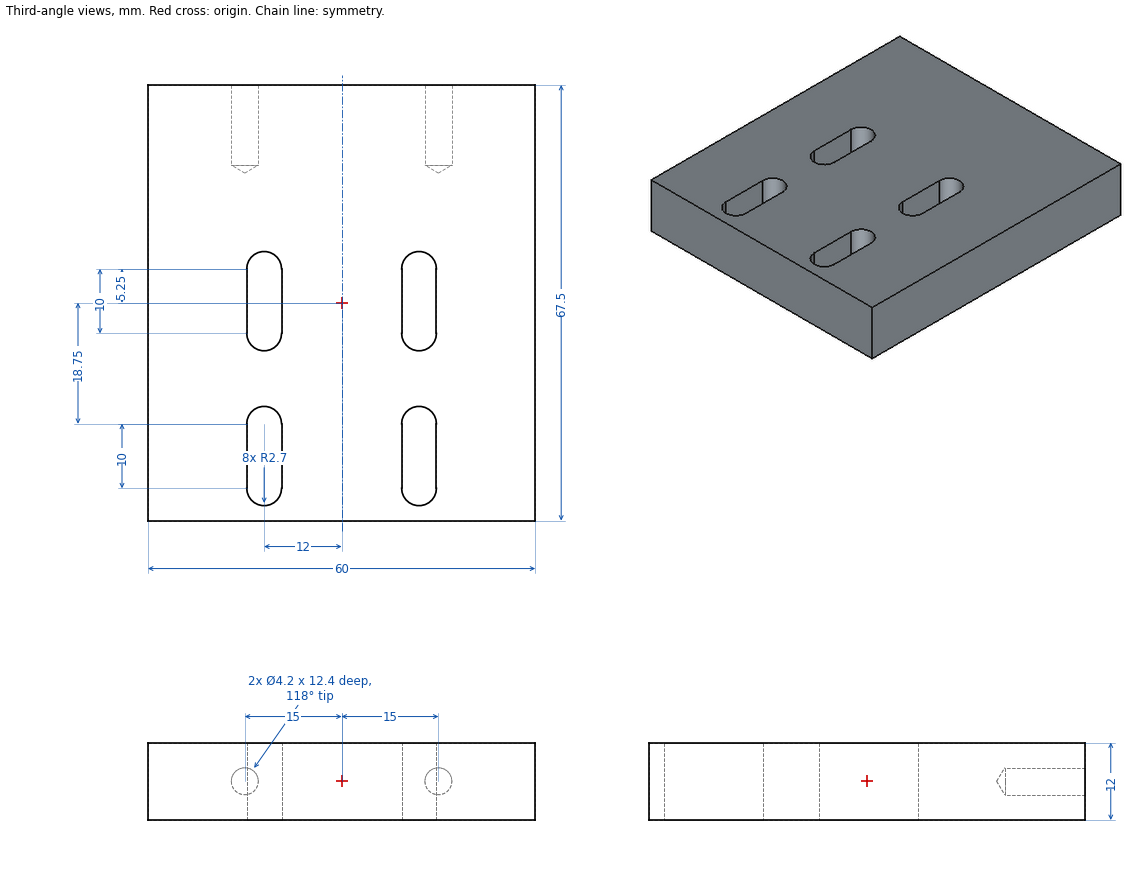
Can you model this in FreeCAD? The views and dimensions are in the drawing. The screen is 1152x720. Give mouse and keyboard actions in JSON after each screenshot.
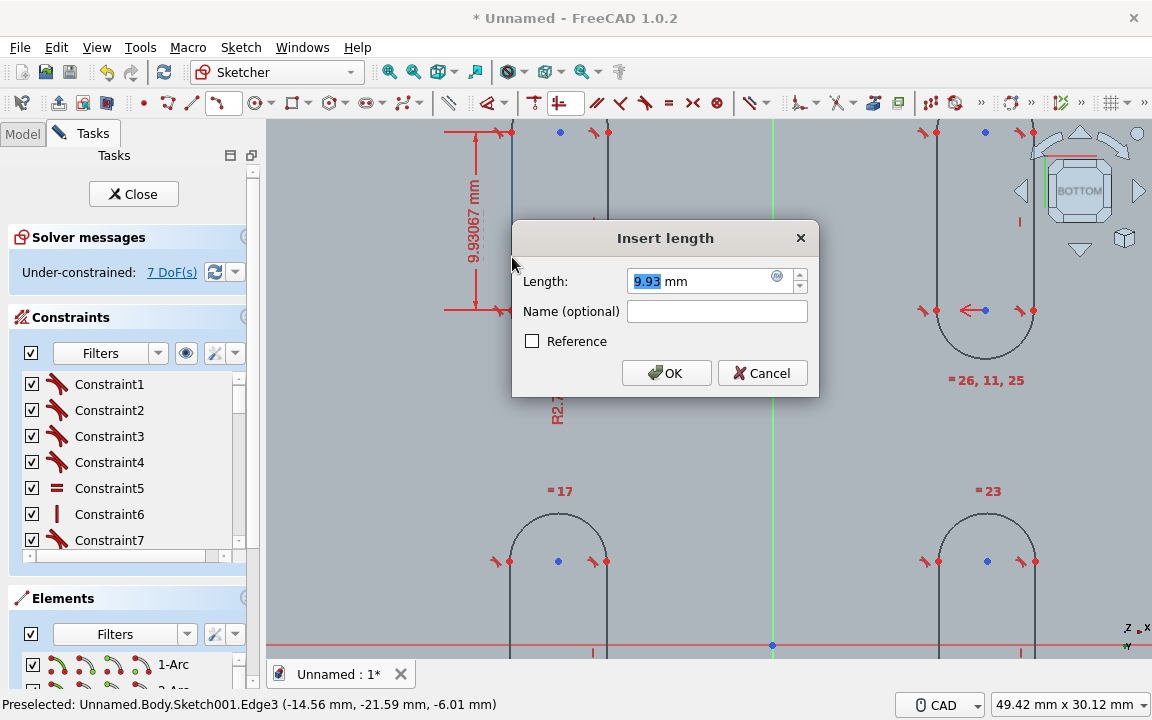
{"action": "type", "text": "10"}
{"action": "key", "text": "Return"}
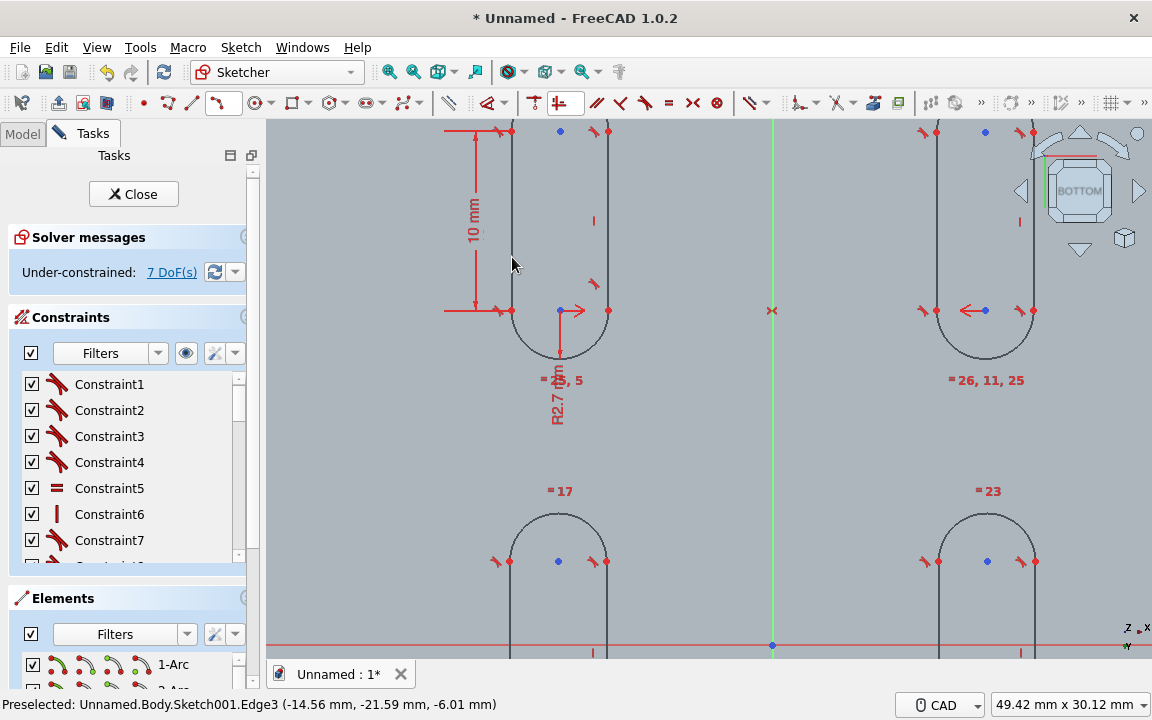
{"action": "left_click", "coordinate": [937, 257]}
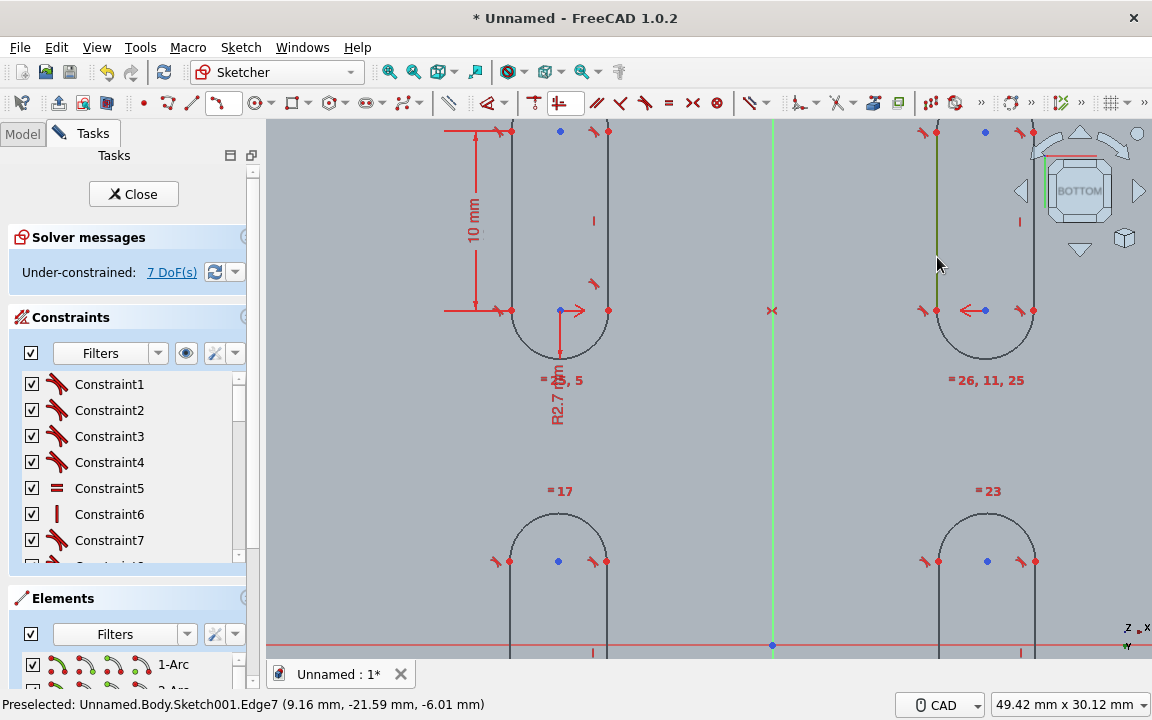
{"action": "key", "text": "i"}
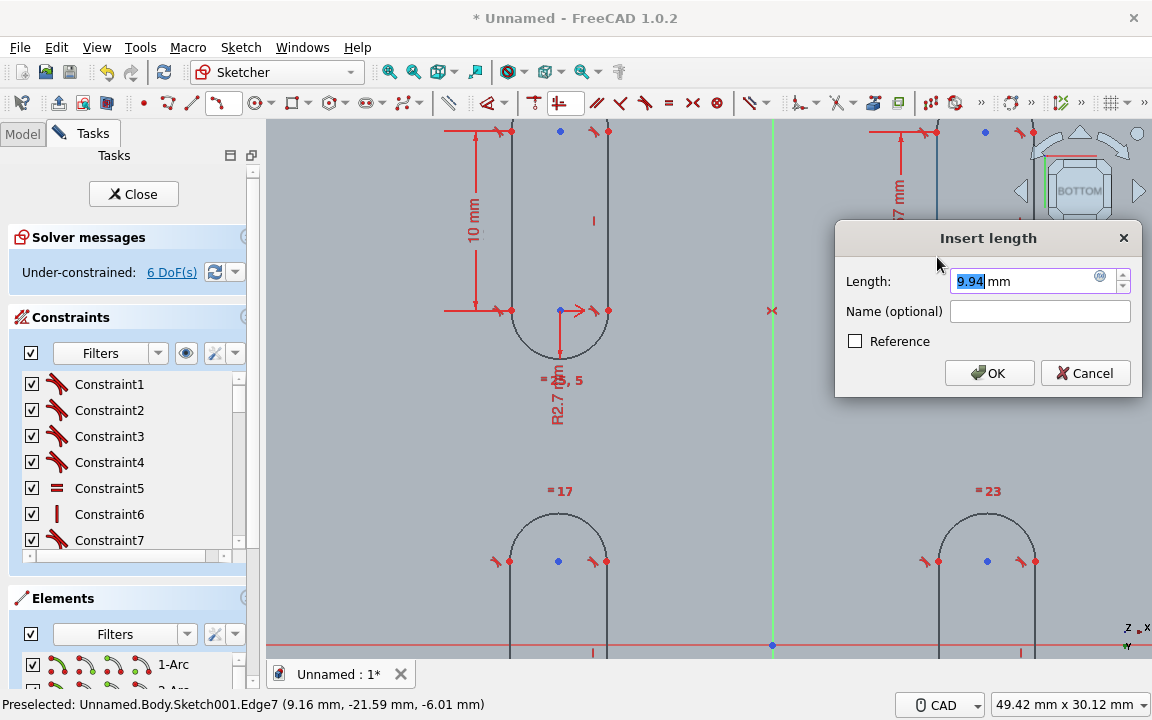
{"action": "type", "text": "10"}
{"action": "key", "text": "Return"}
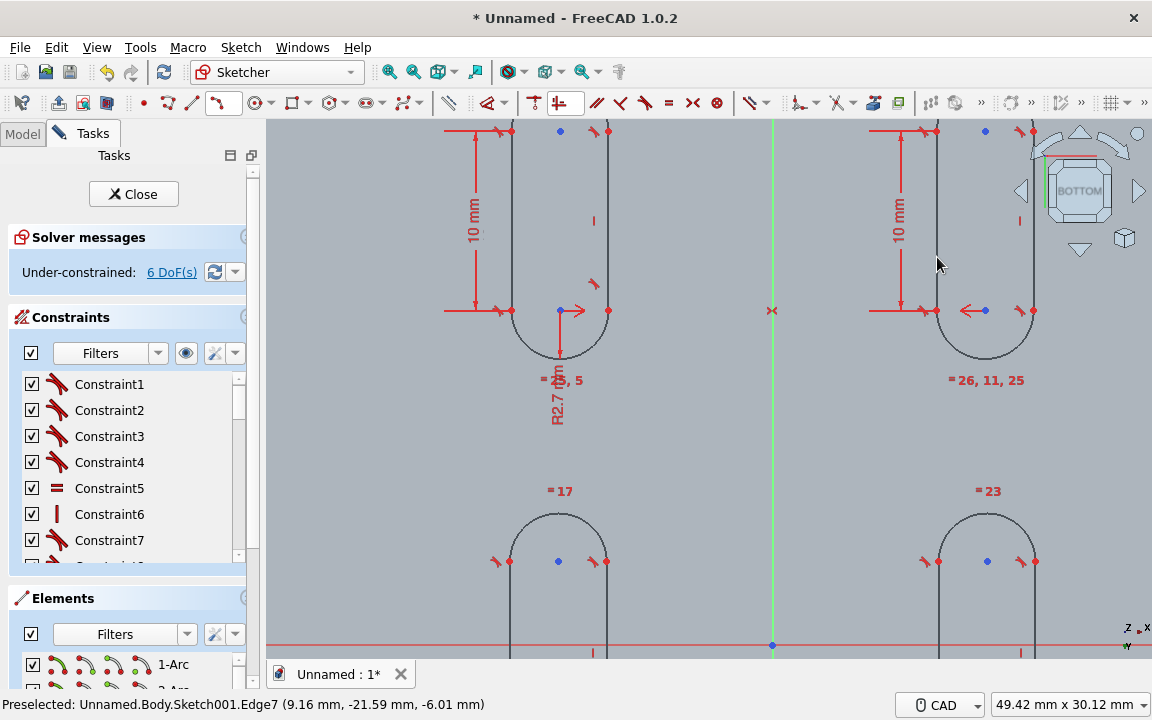
{"action": "left_click", "coordinate": [510, 616]}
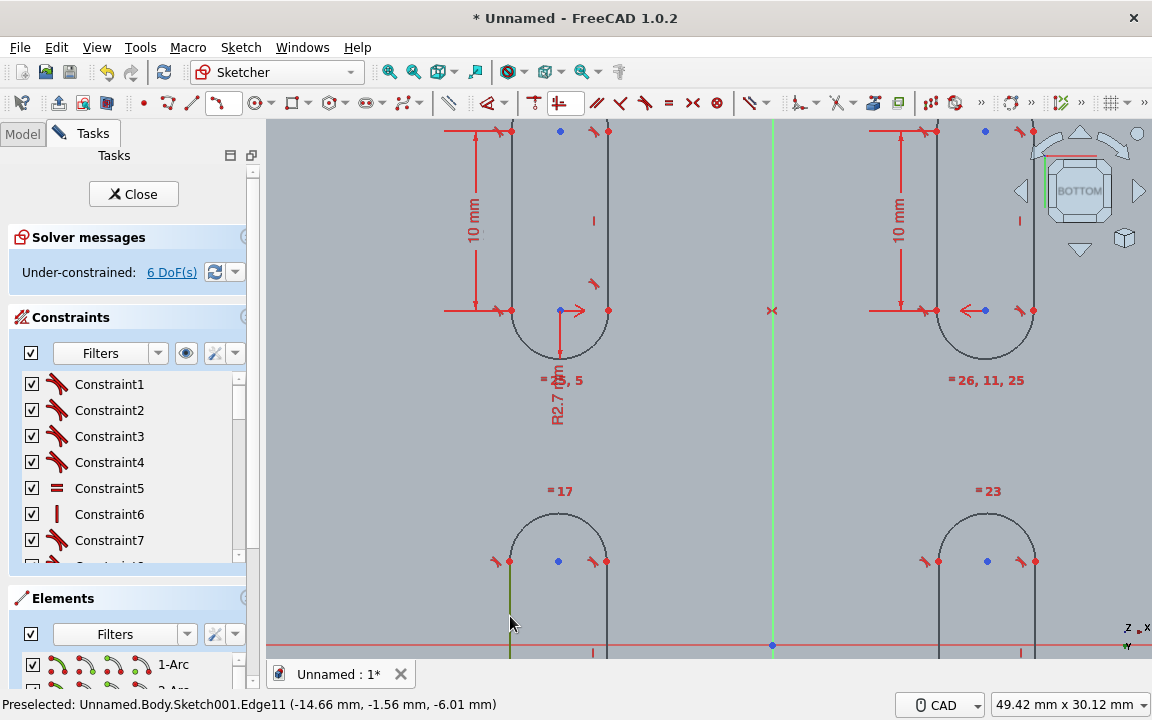
{"action": "left_click", "coordinate": [506, 104]}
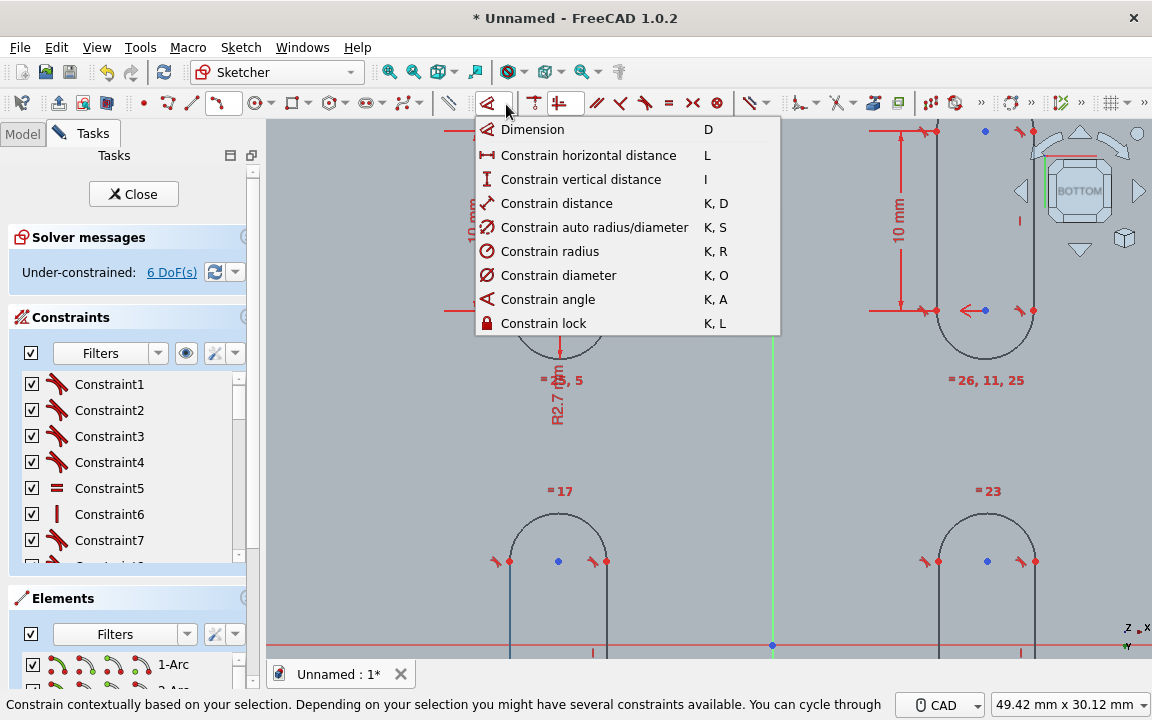
{"action": "left_click", "coordinate": [628, 179]}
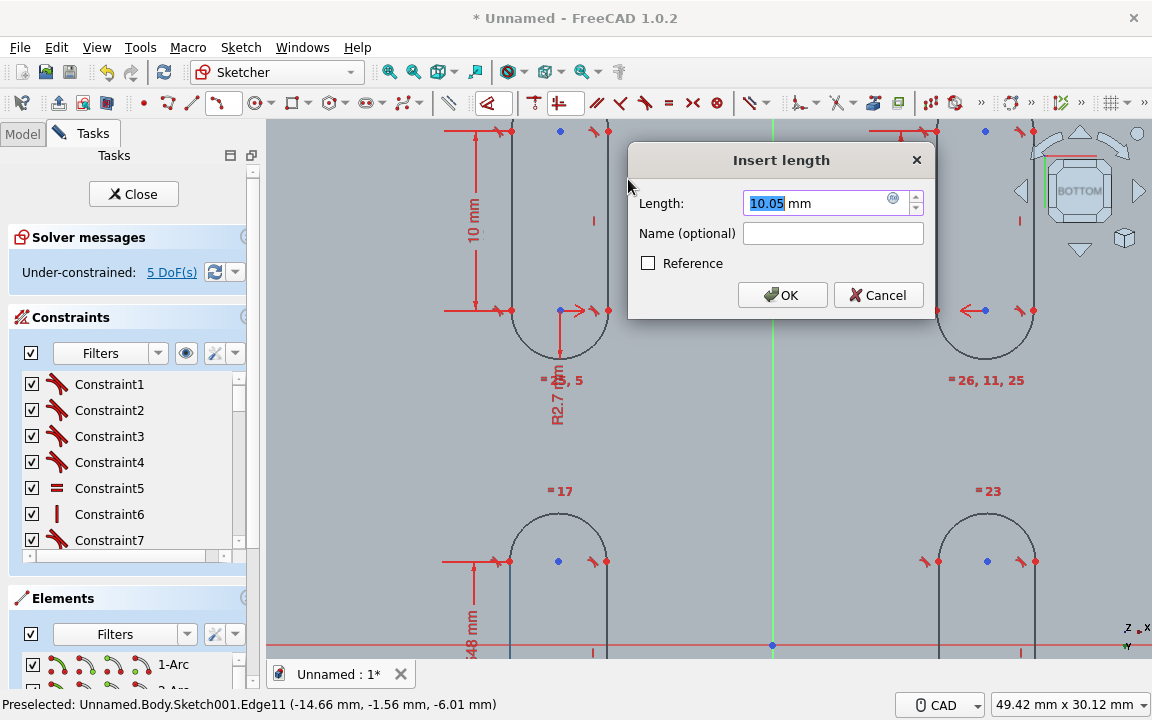
{"action": "type", "text": "10"}
{"action": "key", "text": "Return"}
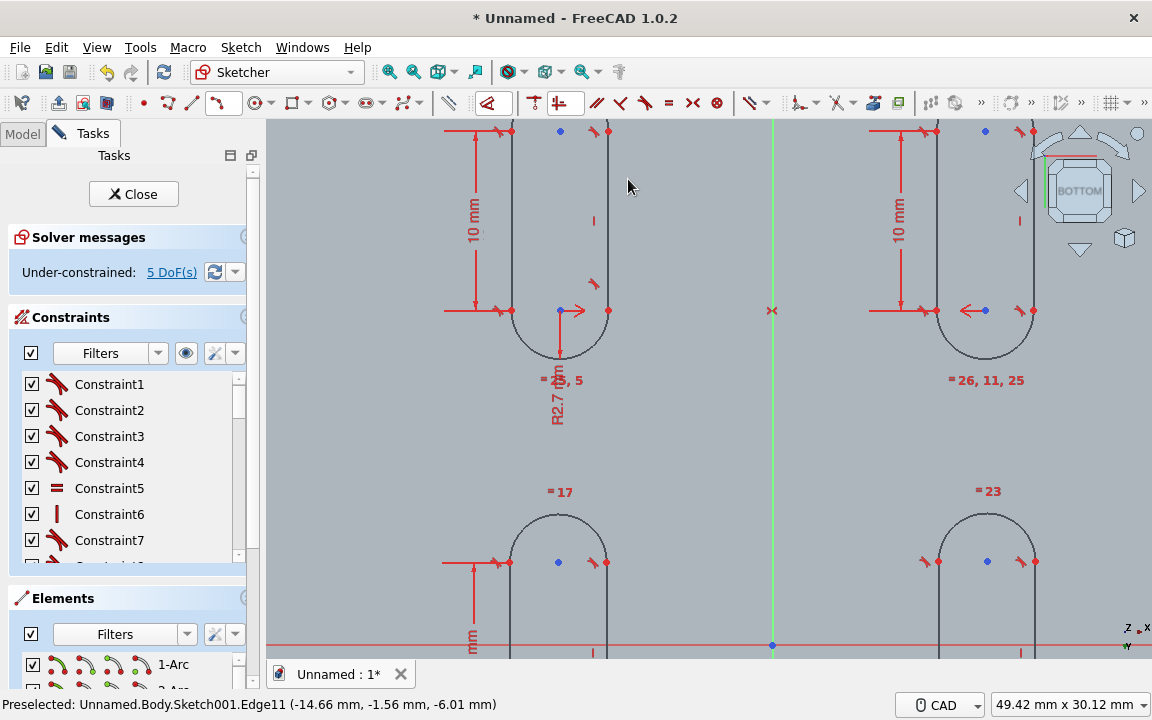
{"action": "left_click", "coordinate": [939, 616]}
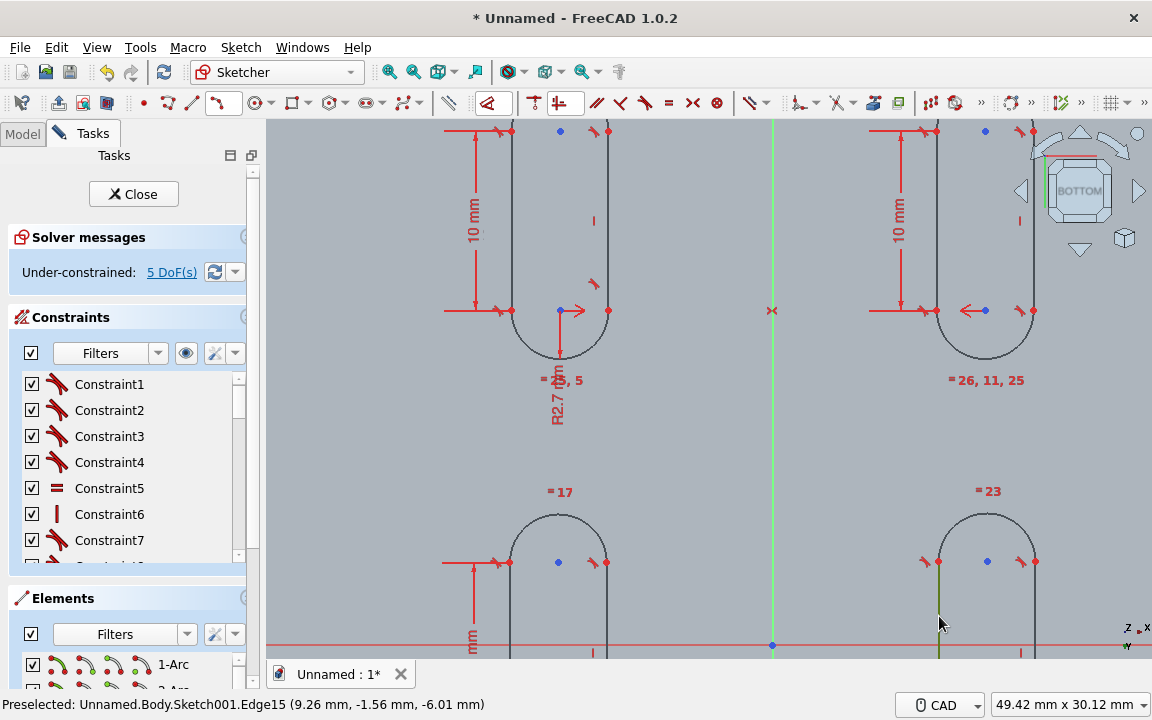
{"action": "key", "text": "i"}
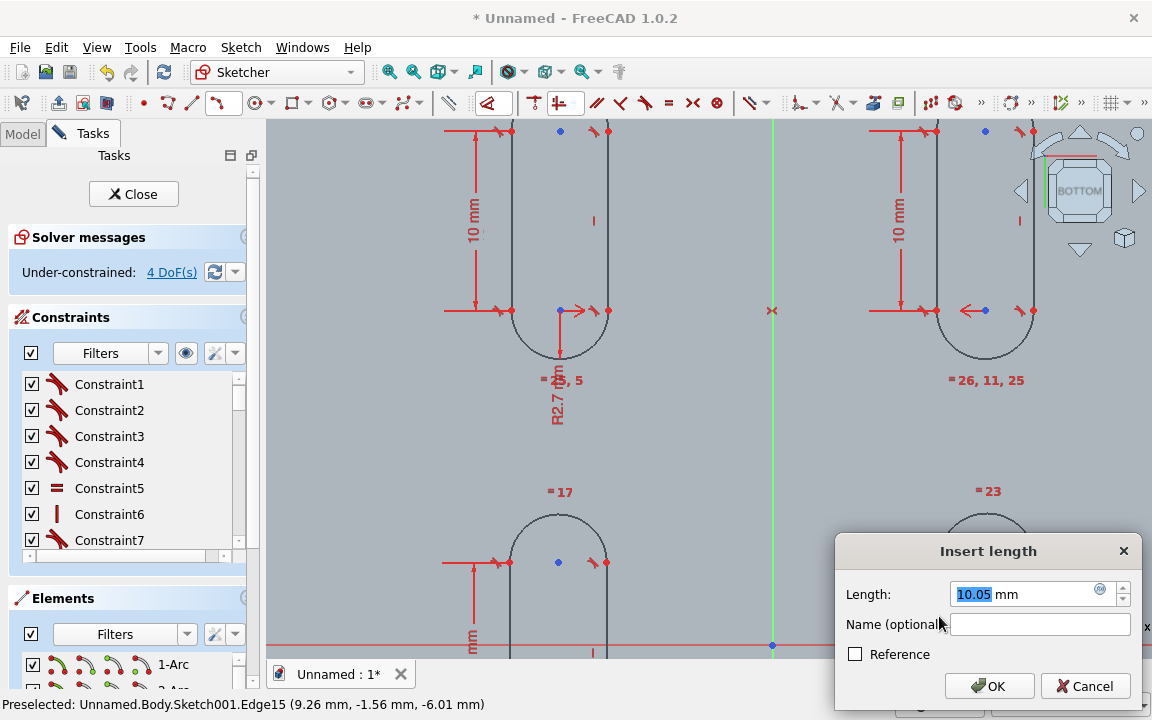
{"action": "type", "text": "10"}
{"action": "key", "text": "Return"}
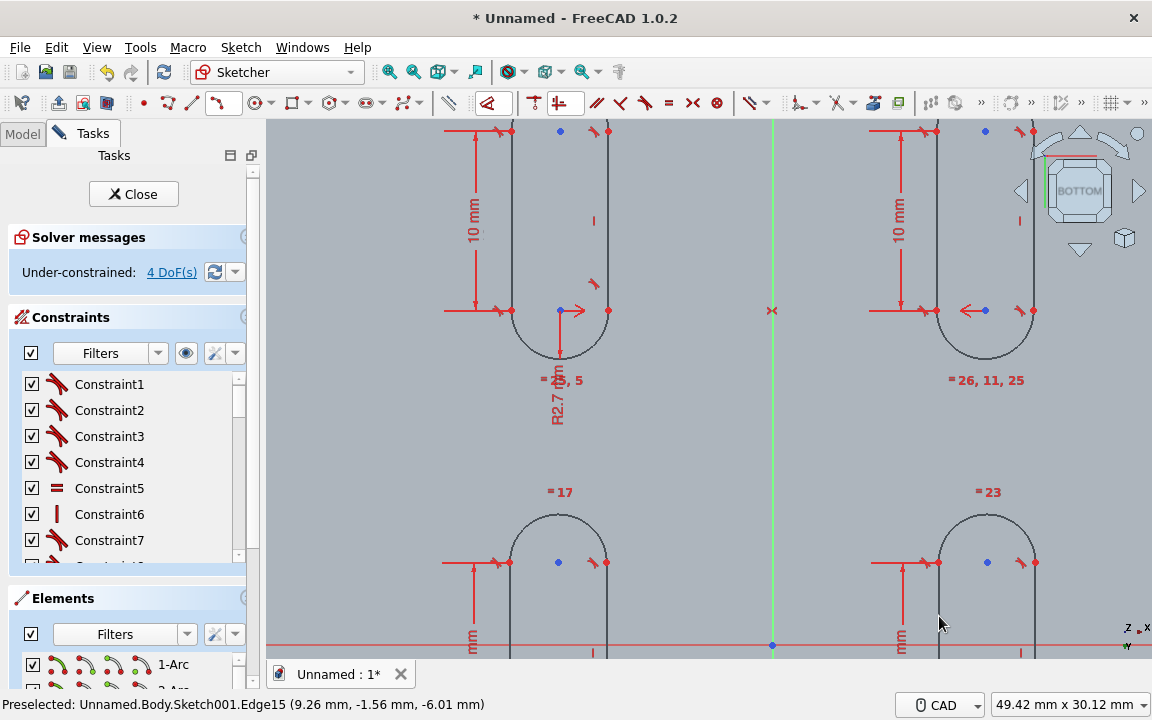
{"action": "left_click", "coordinate": [560, 311]}